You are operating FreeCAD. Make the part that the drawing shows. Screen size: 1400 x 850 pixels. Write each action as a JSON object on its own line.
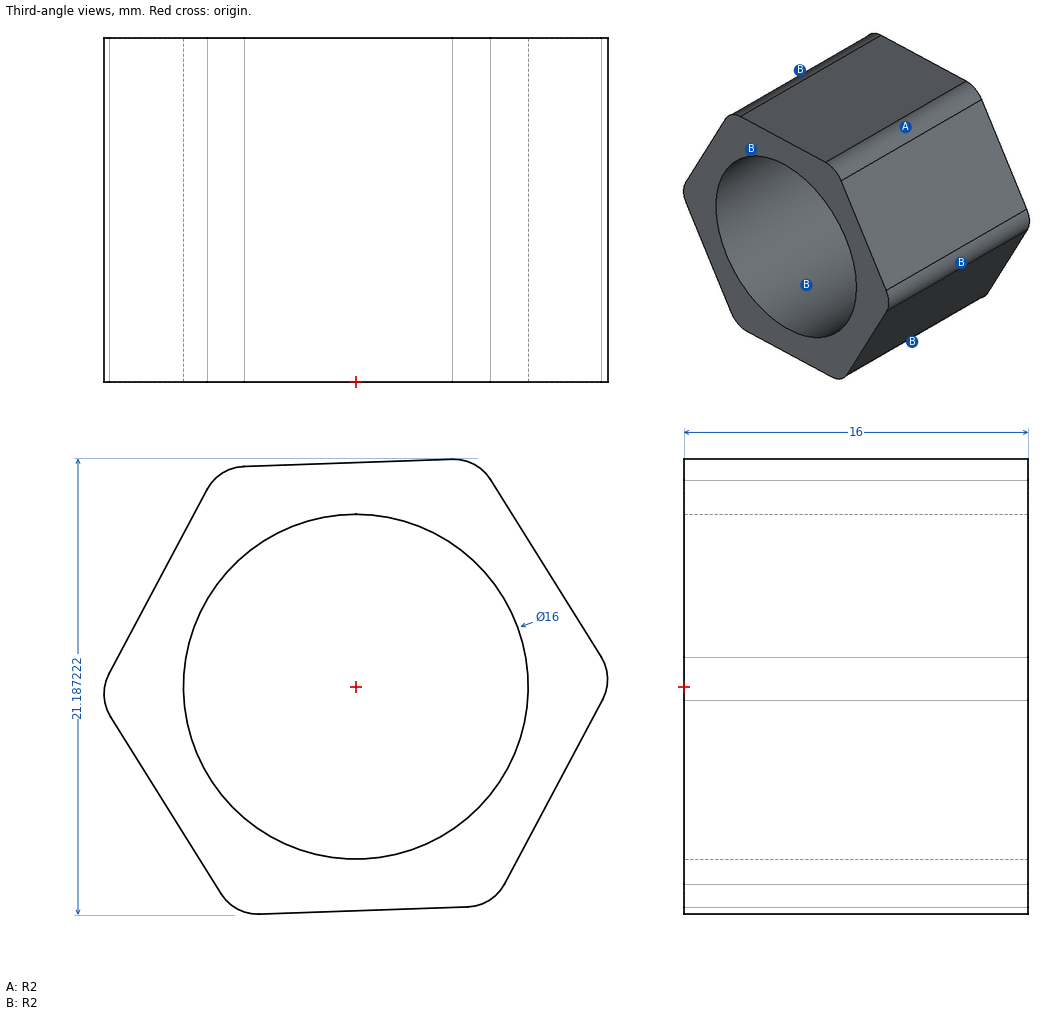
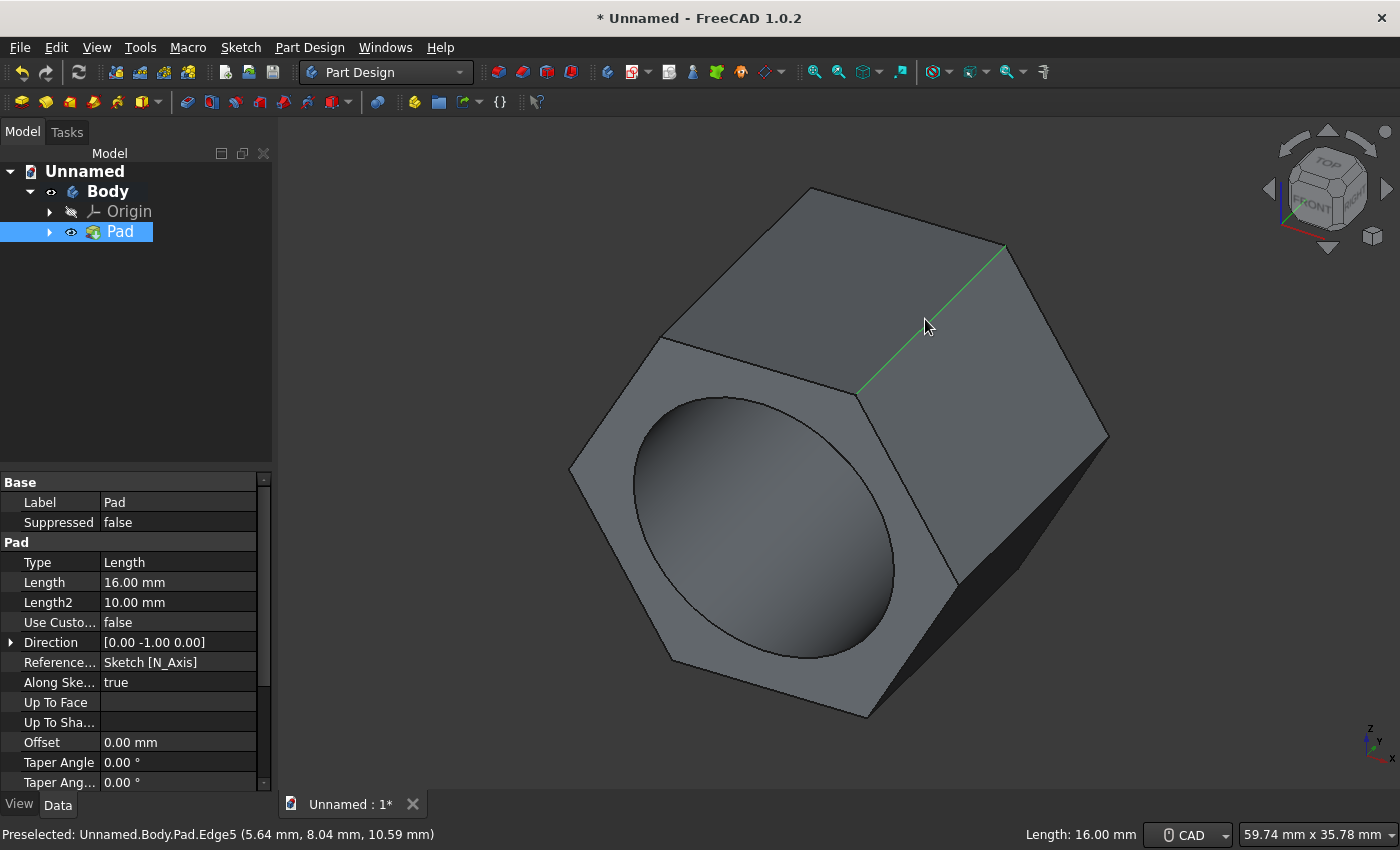
{"action": "left_click", "coordinate": [500, 72]}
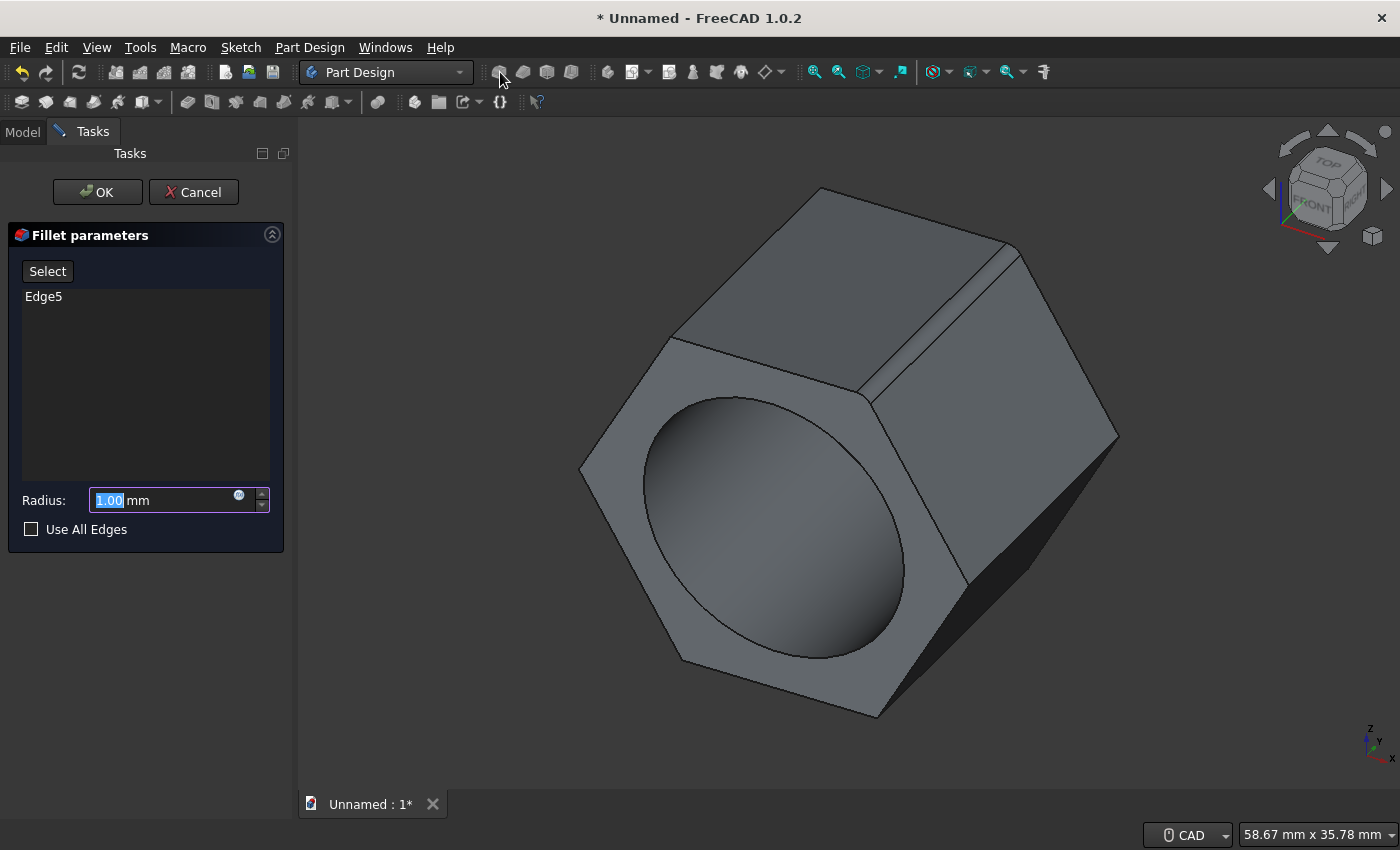
{"action": "type", "text": "2"}
{"action": "key", "text": "Tab"}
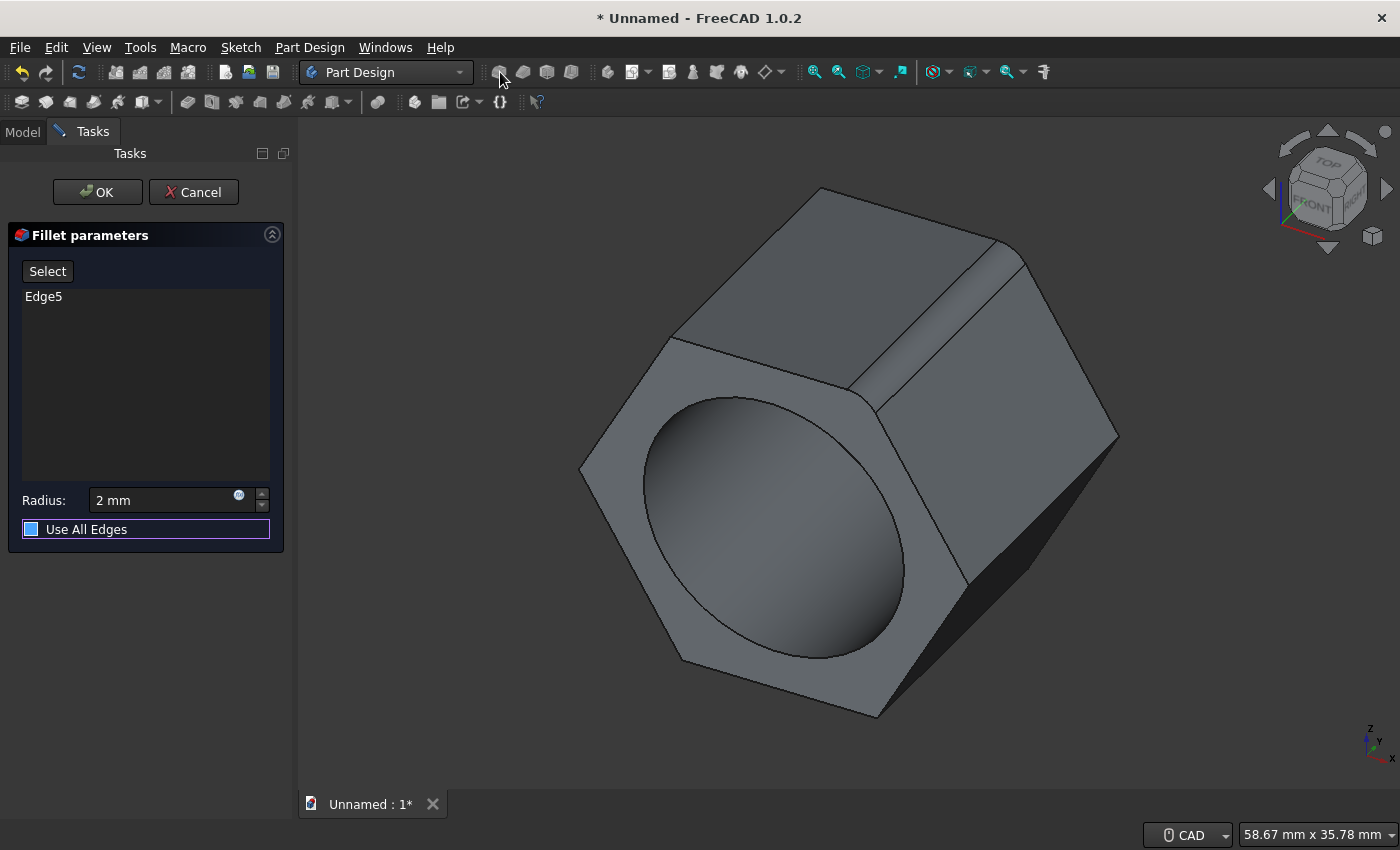
{"action": "left_click", "coordinate": [98, 192]}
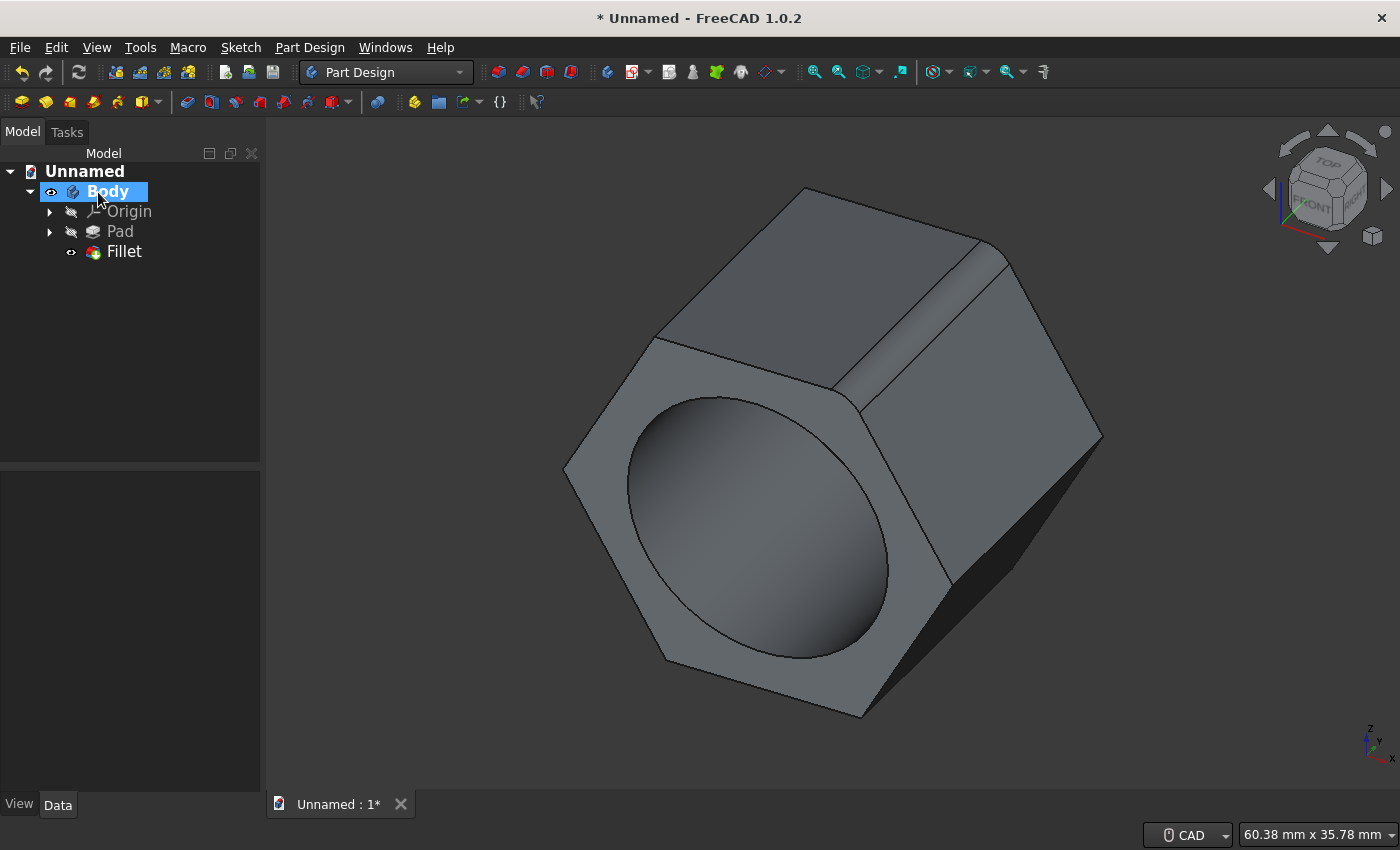
{"action": "key", "text": "0"}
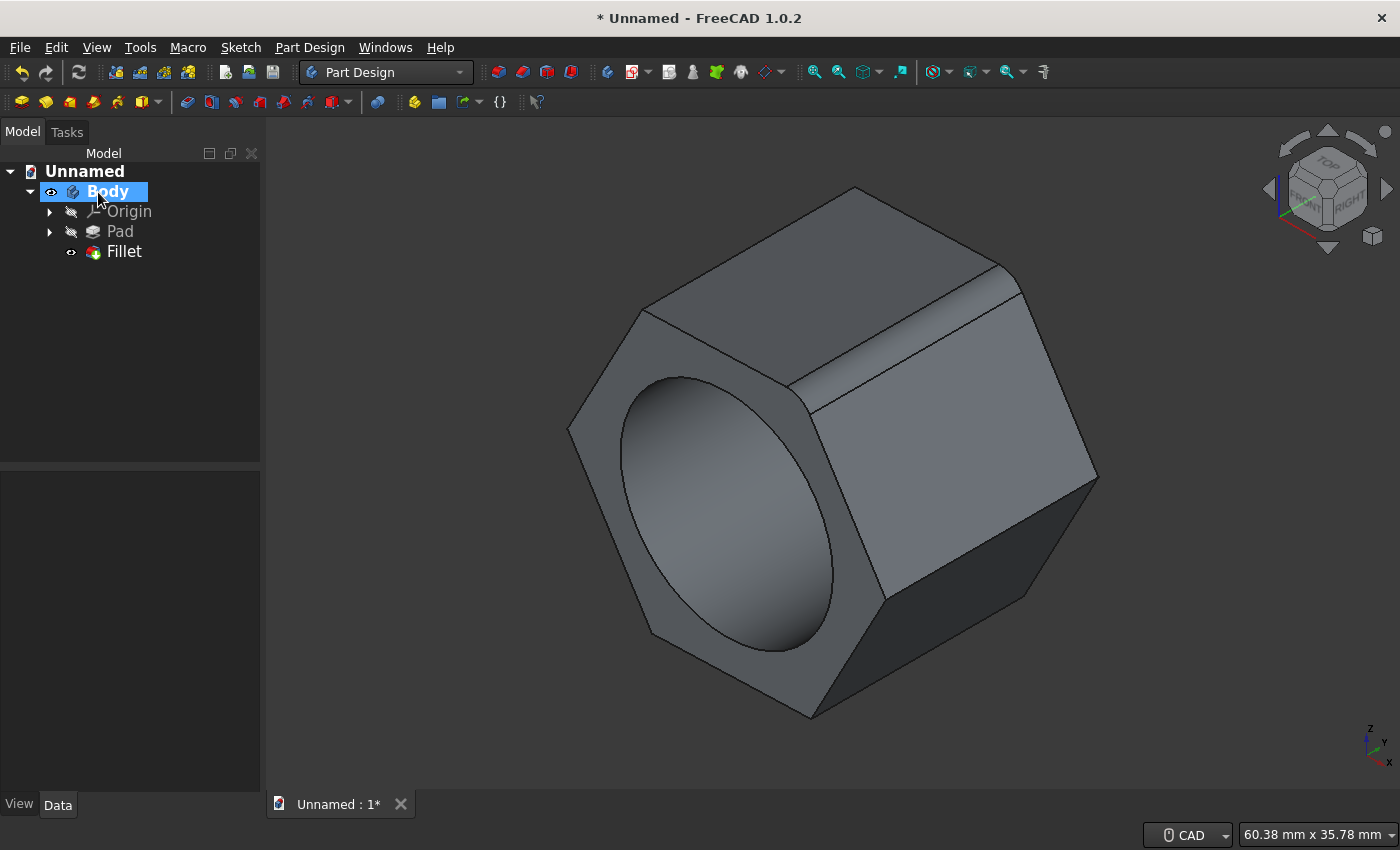
{"action": "key", "text": "2"}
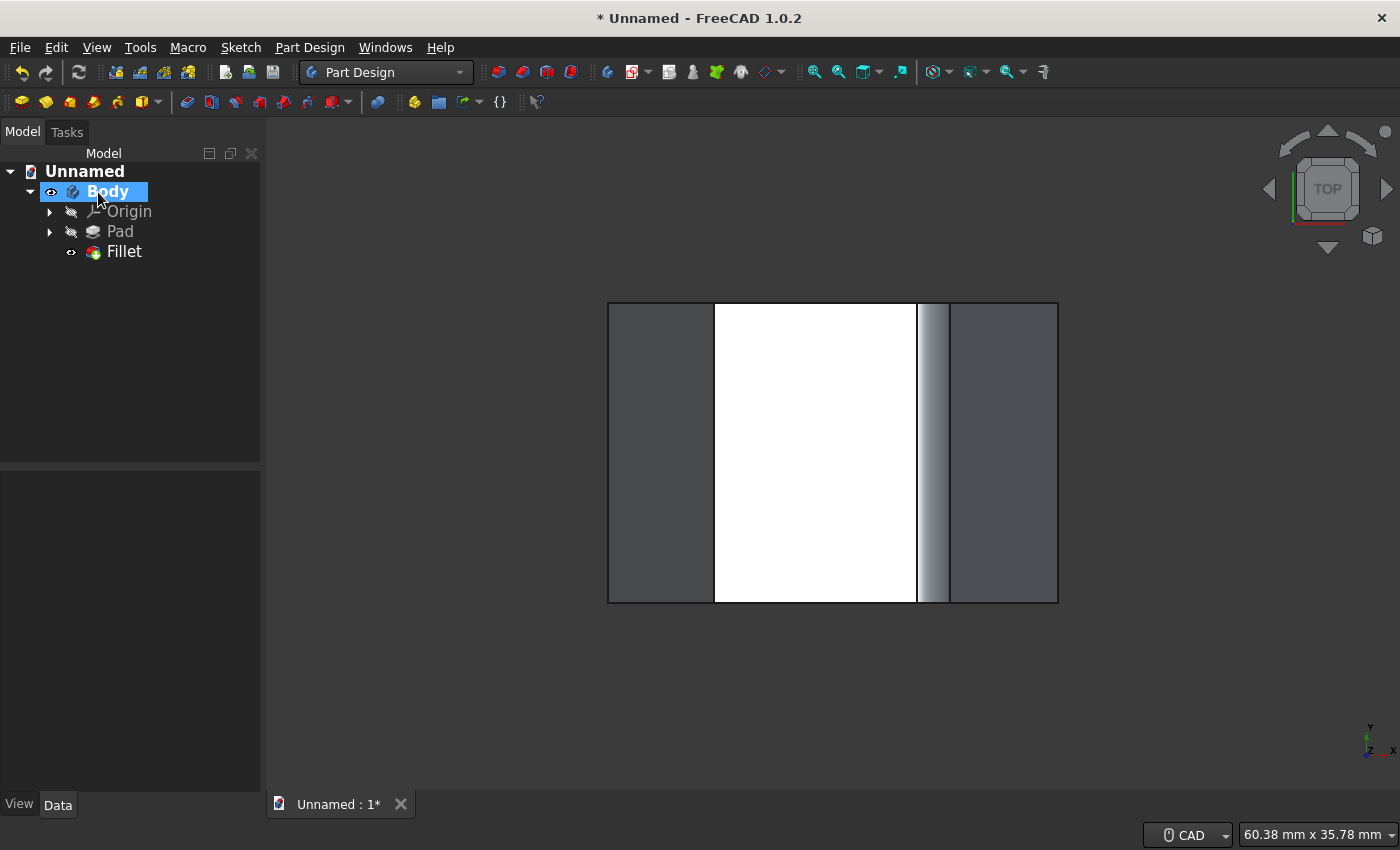
{"action": "left_click", "coordinate": [816, 72]}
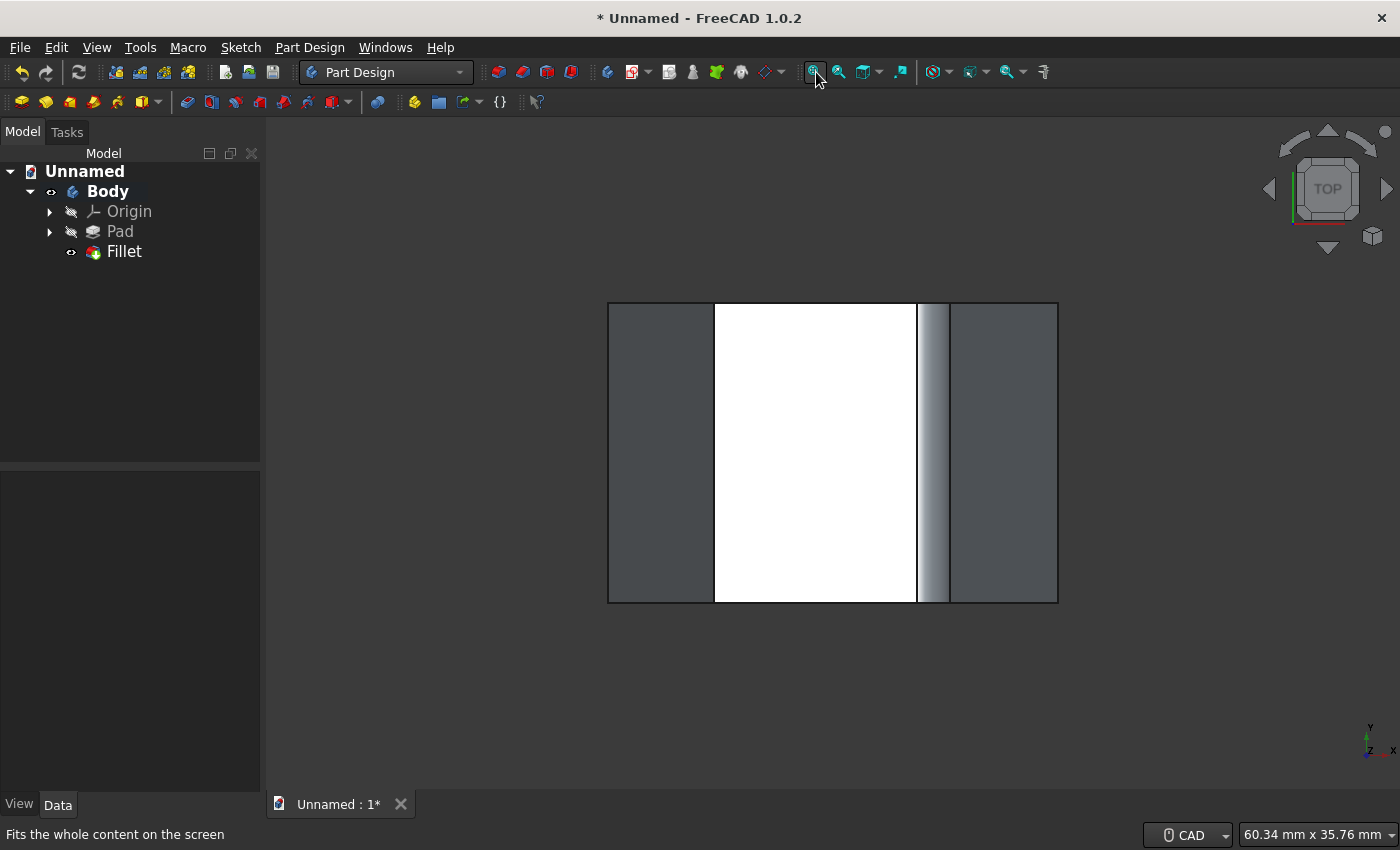
{"action": "key", "text": "1"}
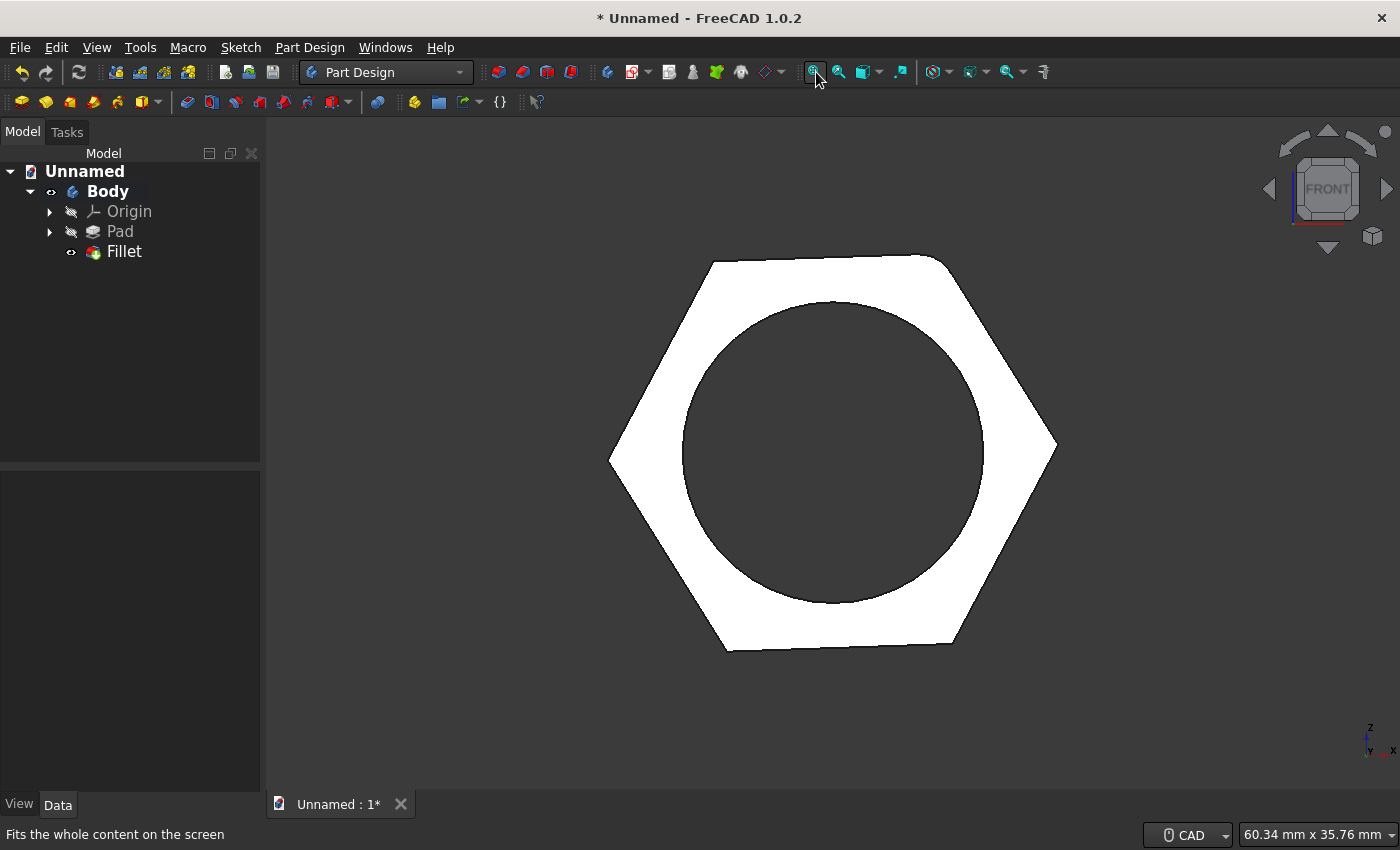
{"action": "key", "text": "3"}